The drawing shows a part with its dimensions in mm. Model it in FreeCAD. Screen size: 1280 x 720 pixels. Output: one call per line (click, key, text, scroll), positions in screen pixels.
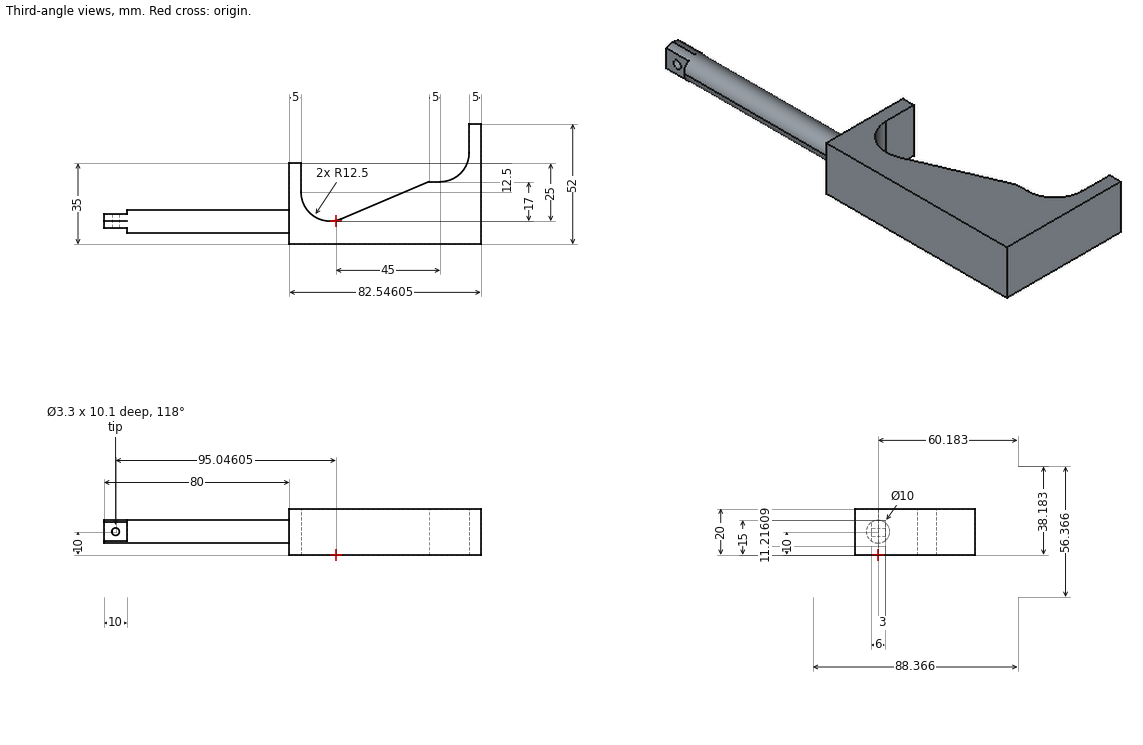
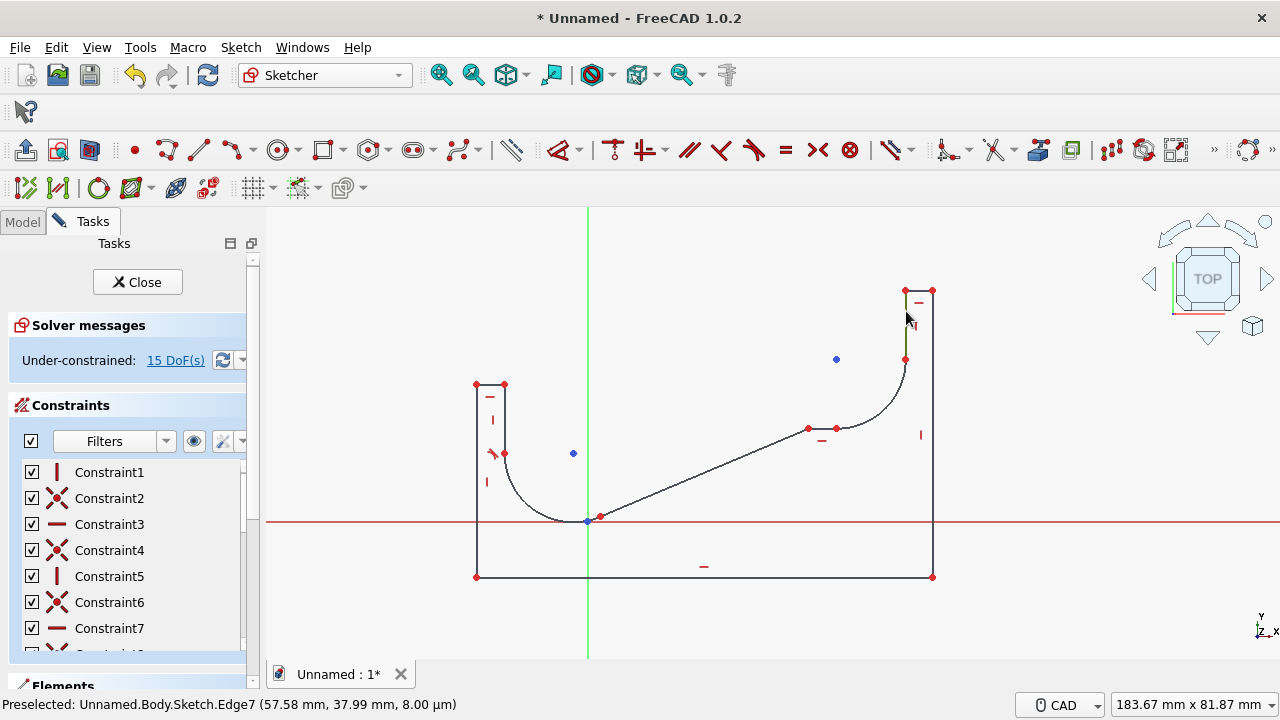
click(868, 421)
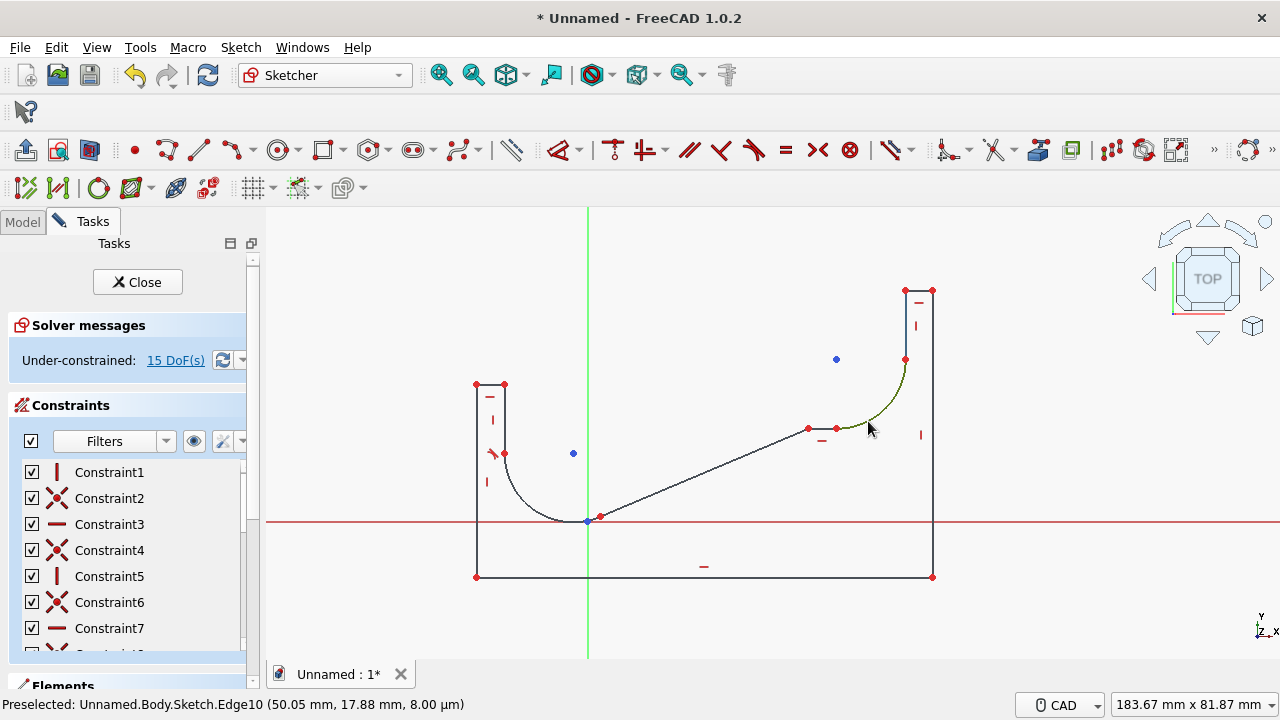
click(754, 150)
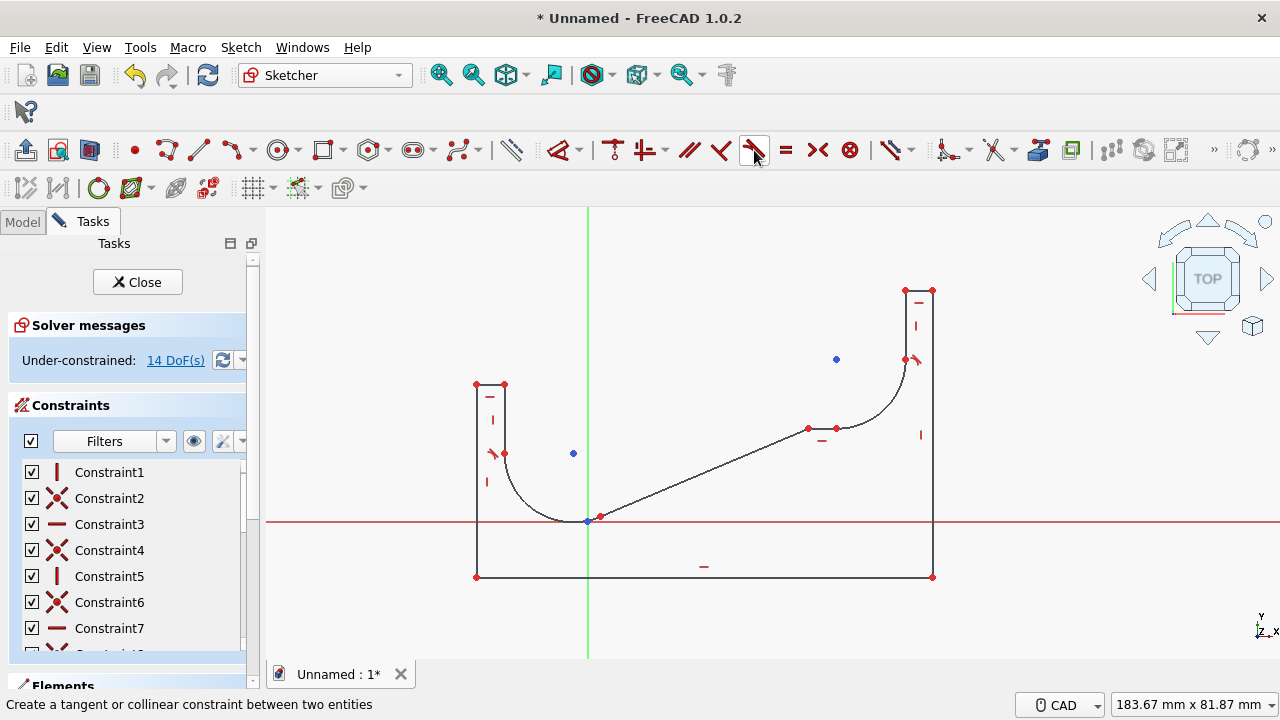
scroll(825, 429, up, 2)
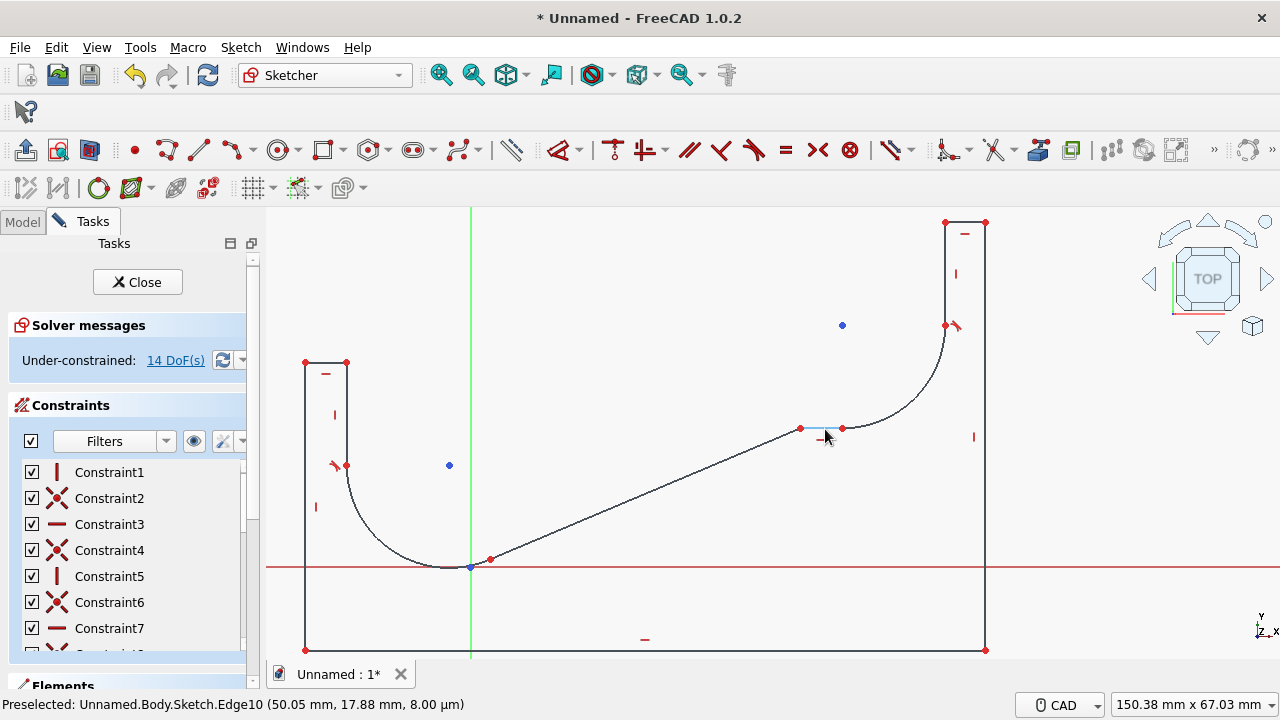
click(825, 428)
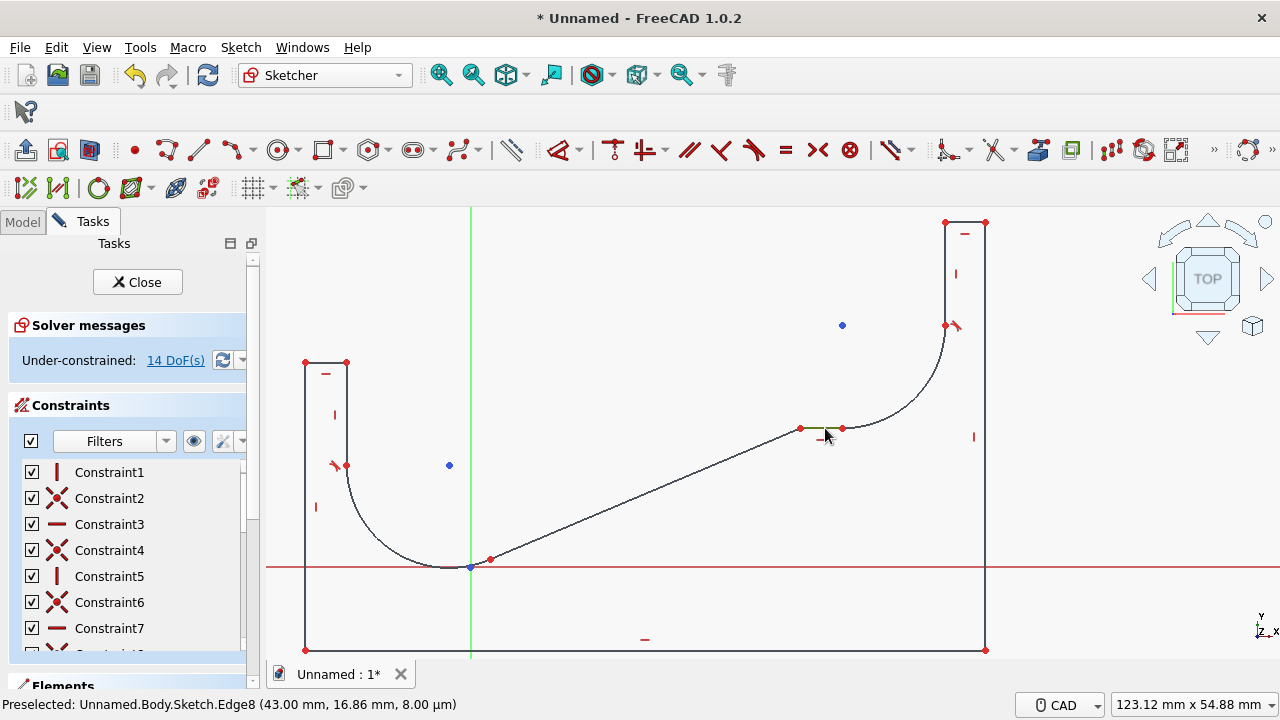
click(889, 417)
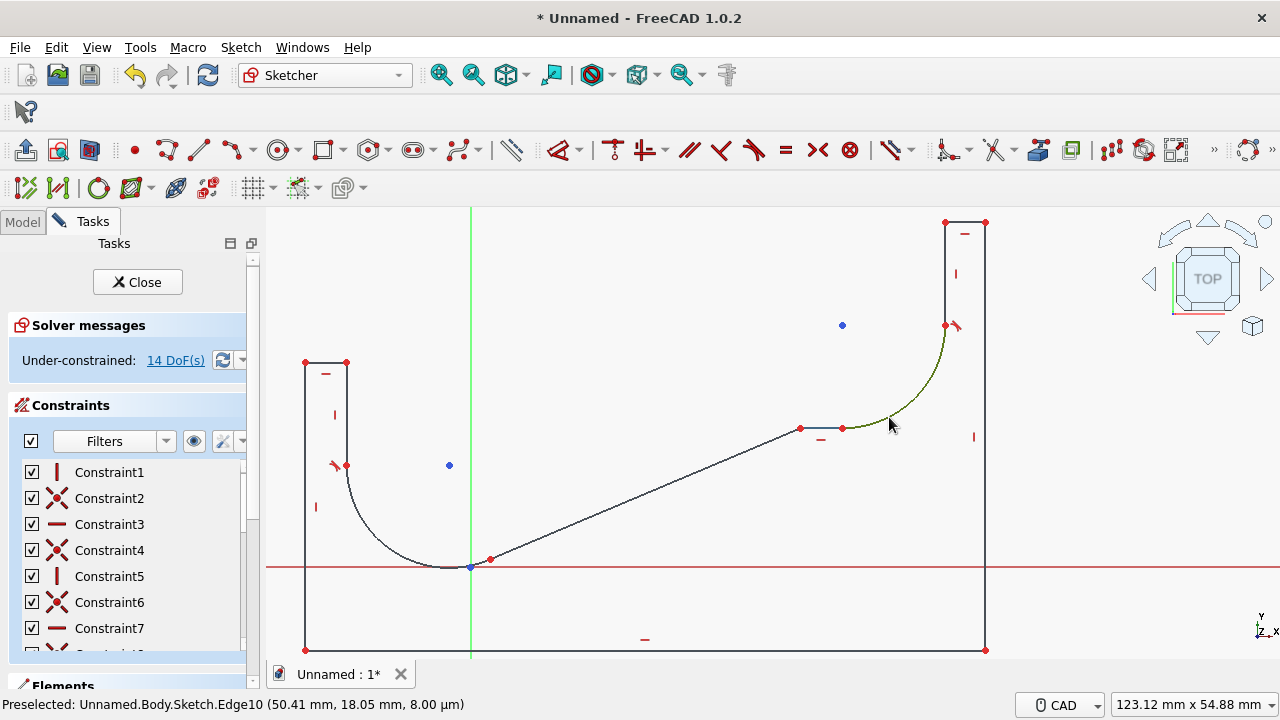
click(754, 150)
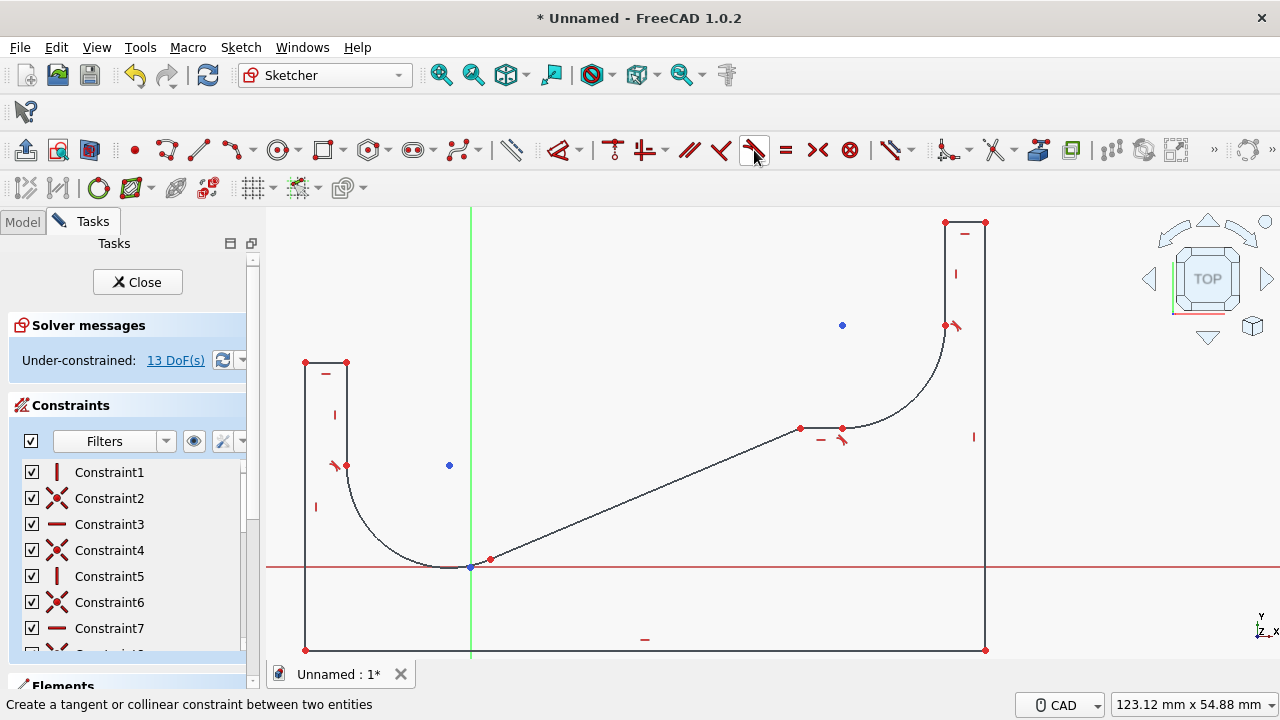
click(707, 468)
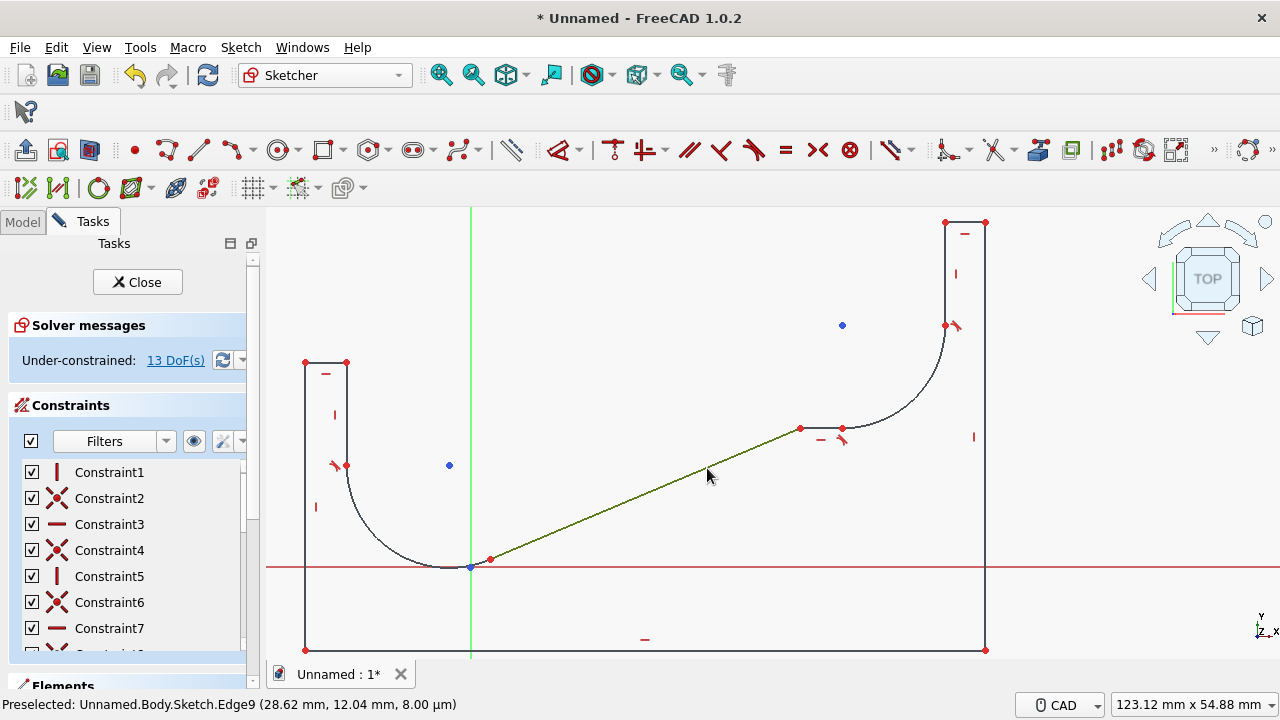
click(364, 523)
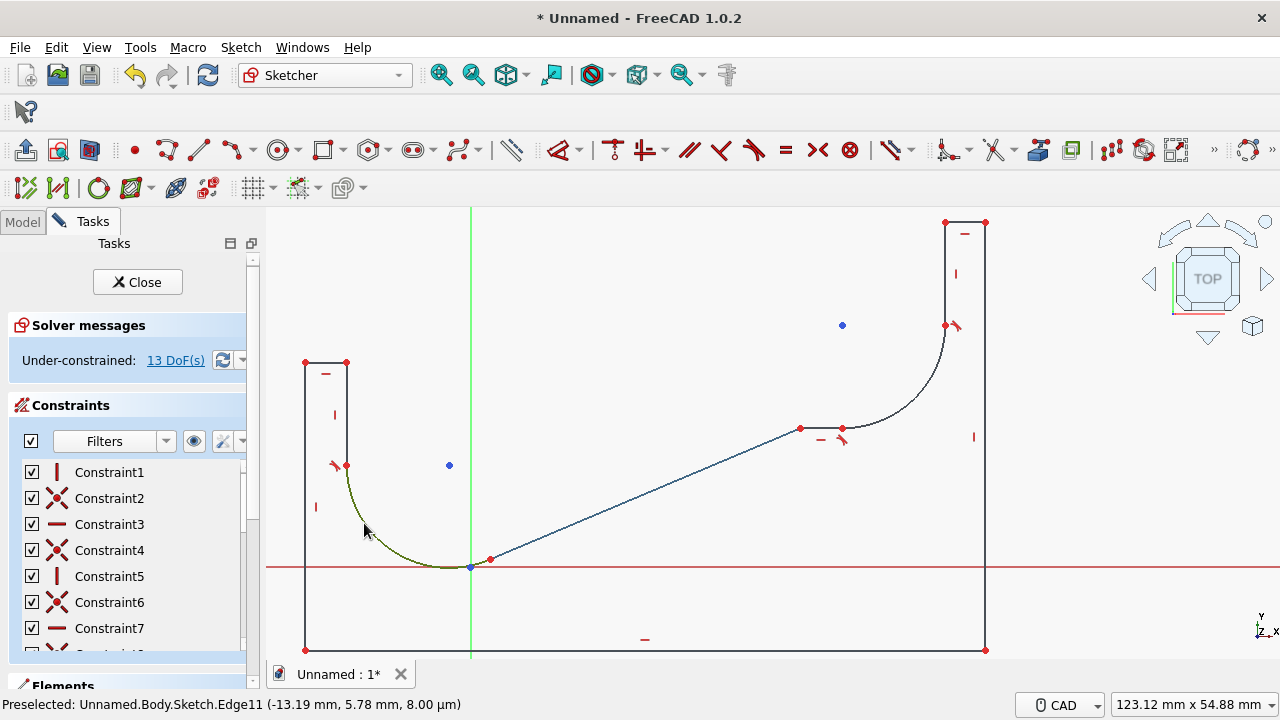
click(754, 150)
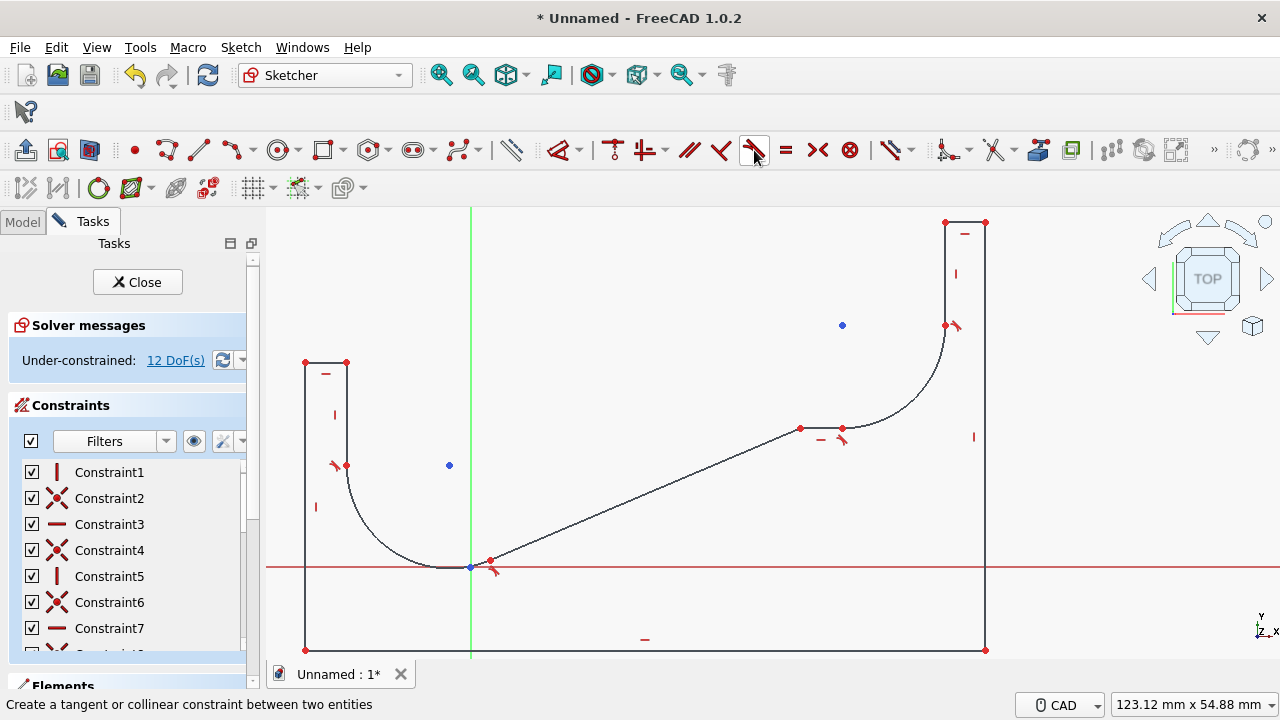
click(889, 417)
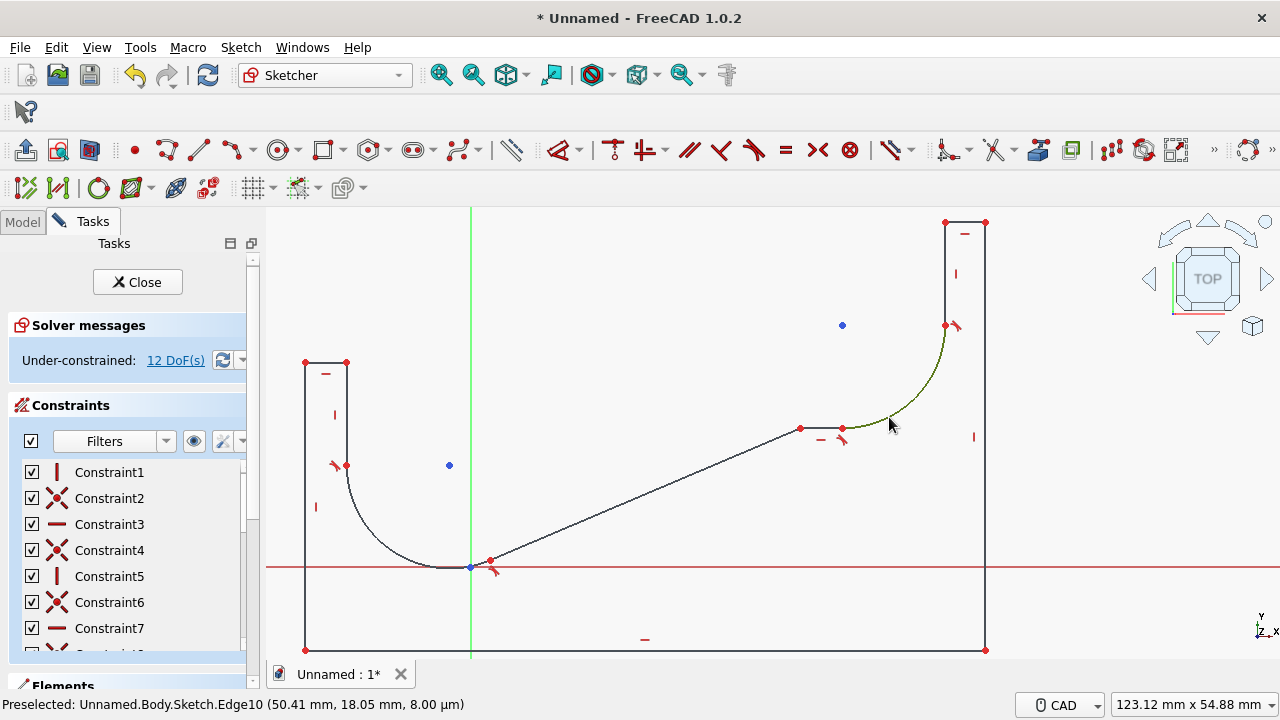
click(364, 523)